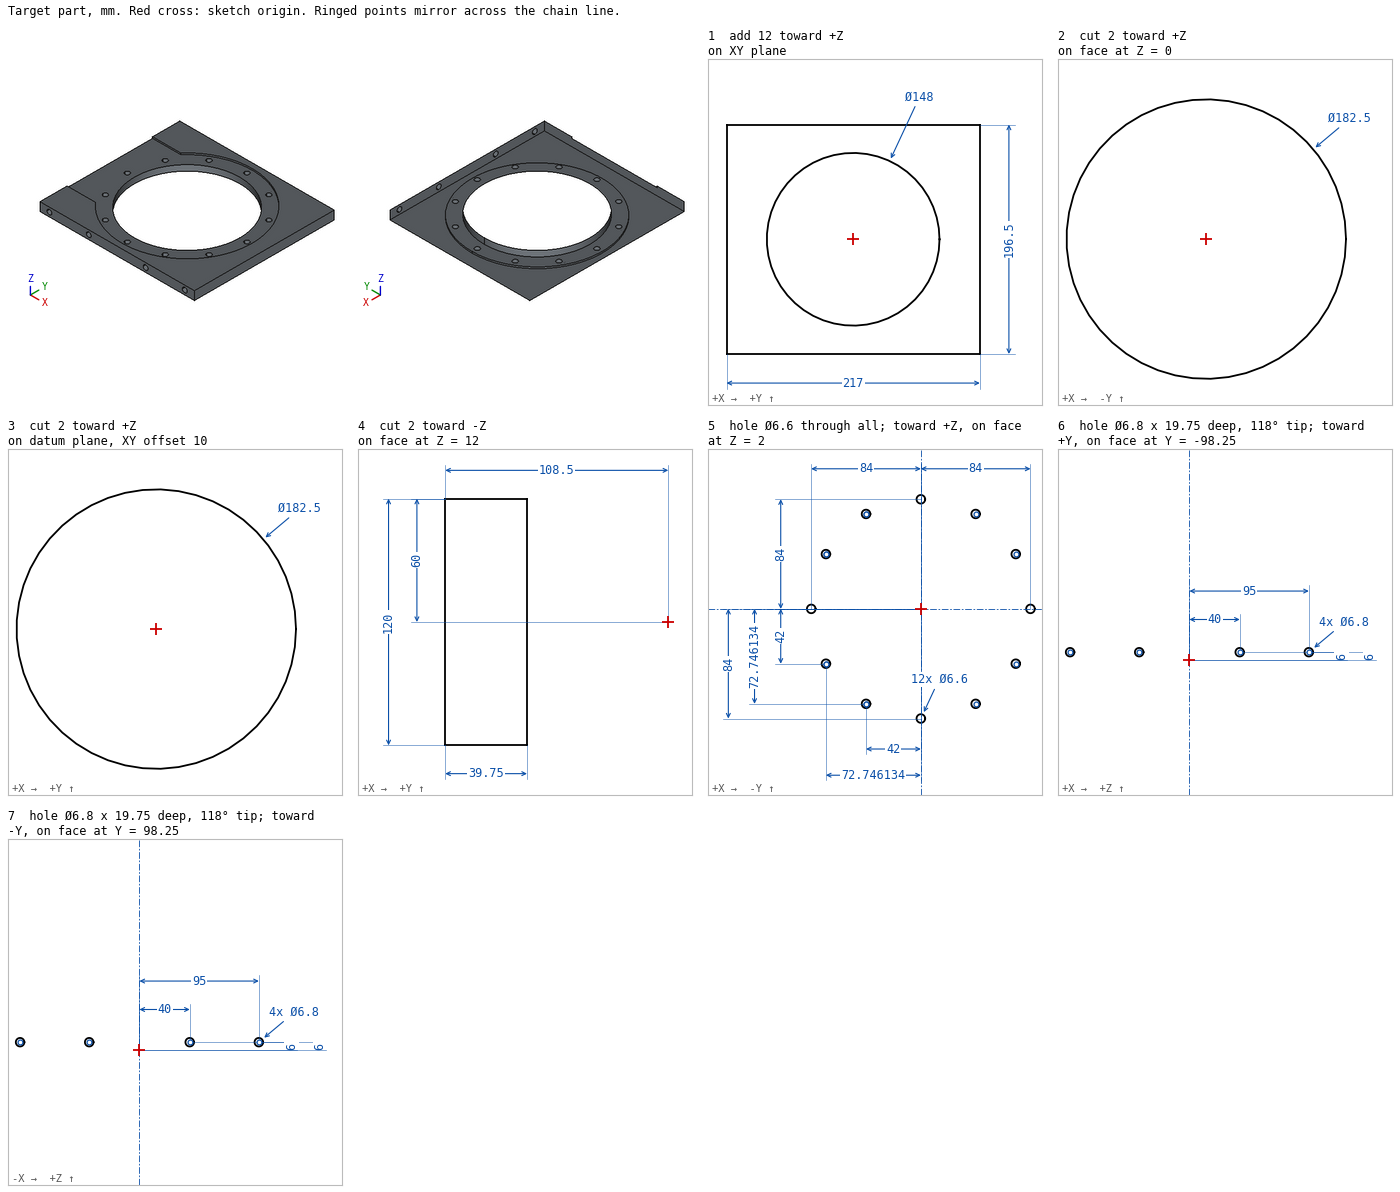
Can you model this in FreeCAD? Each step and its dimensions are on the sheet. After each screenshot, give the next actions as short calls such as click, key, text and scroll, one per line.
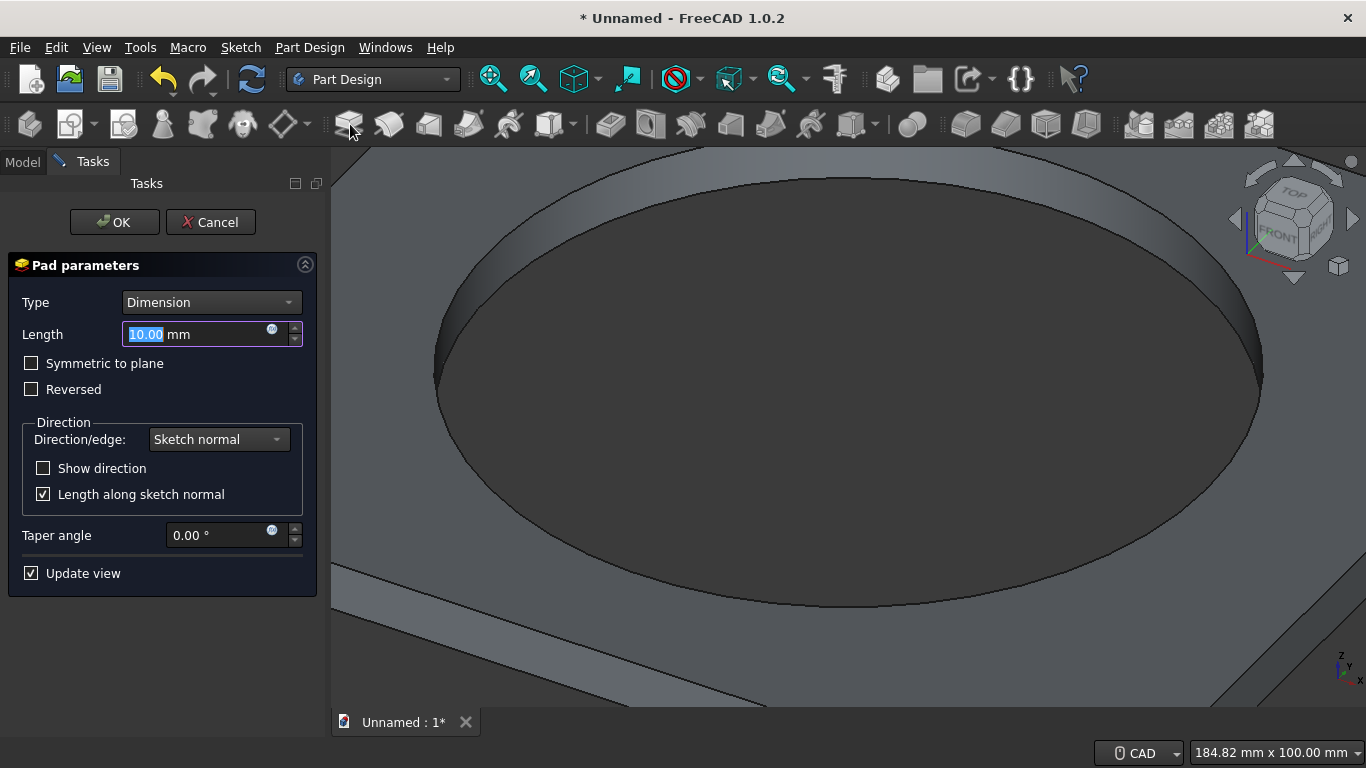
text(12)
key(Tab)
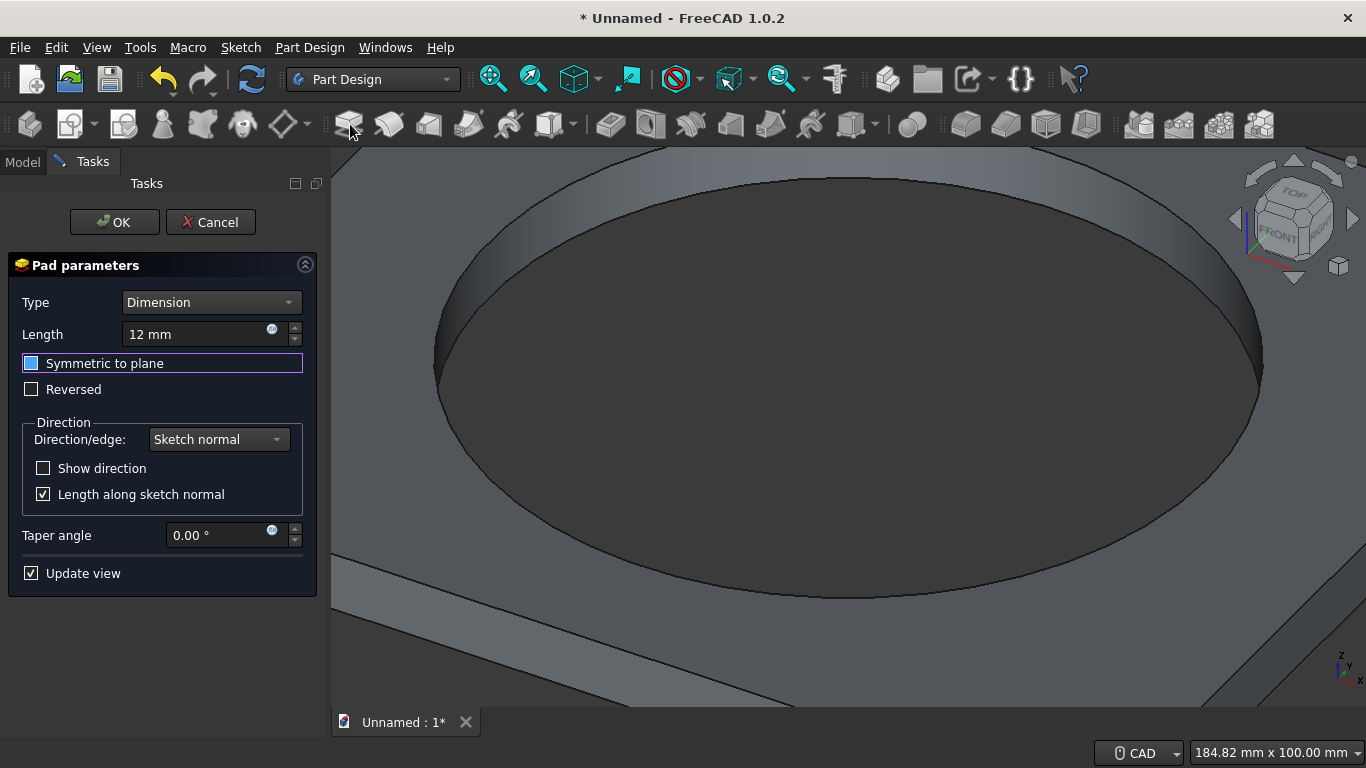
click(115, 222)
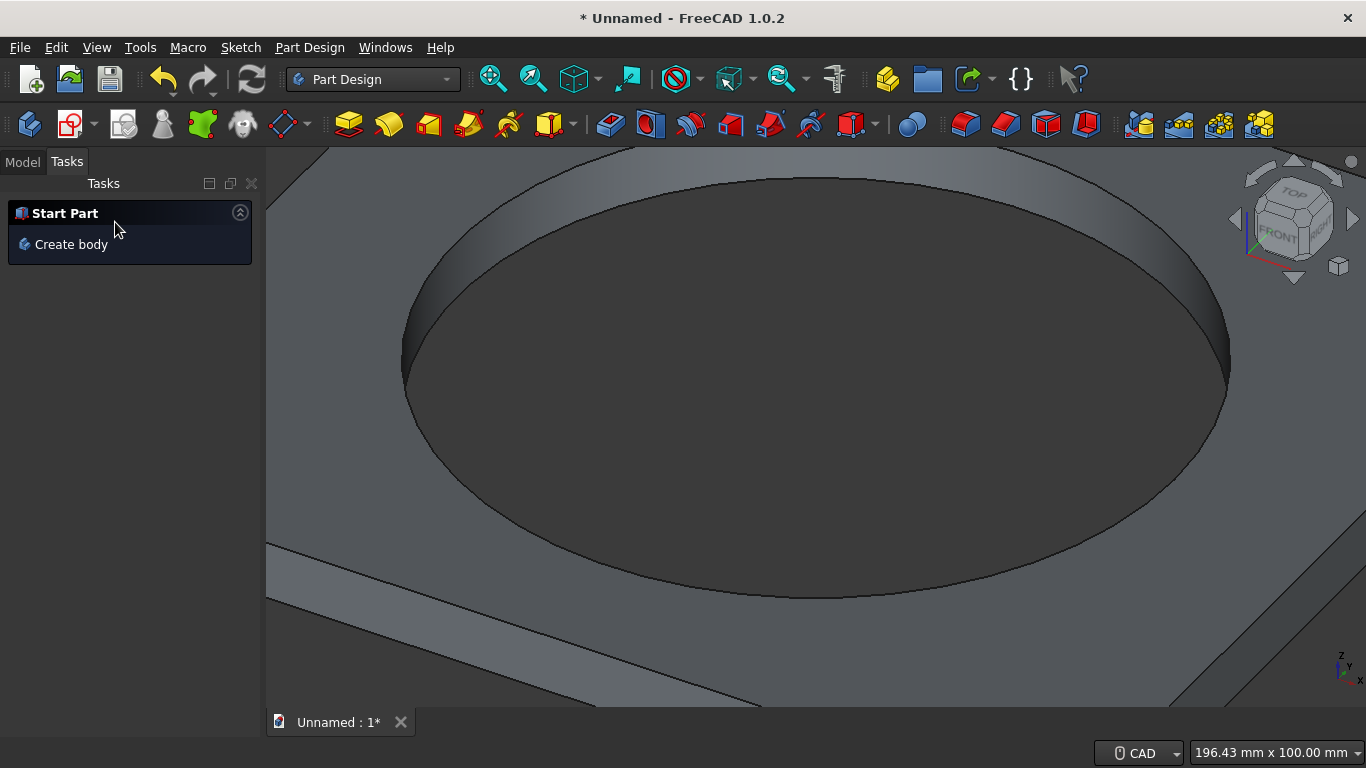
click(494, 80)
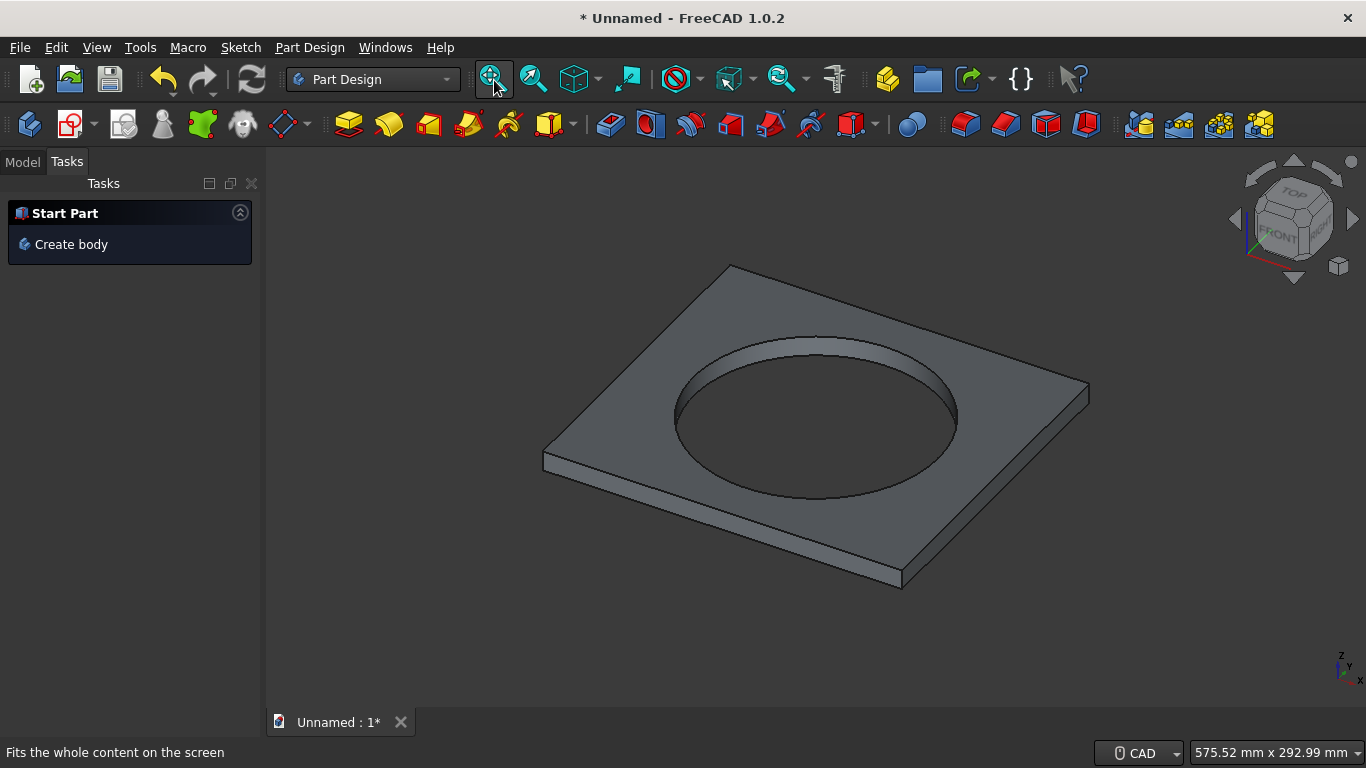
key(5)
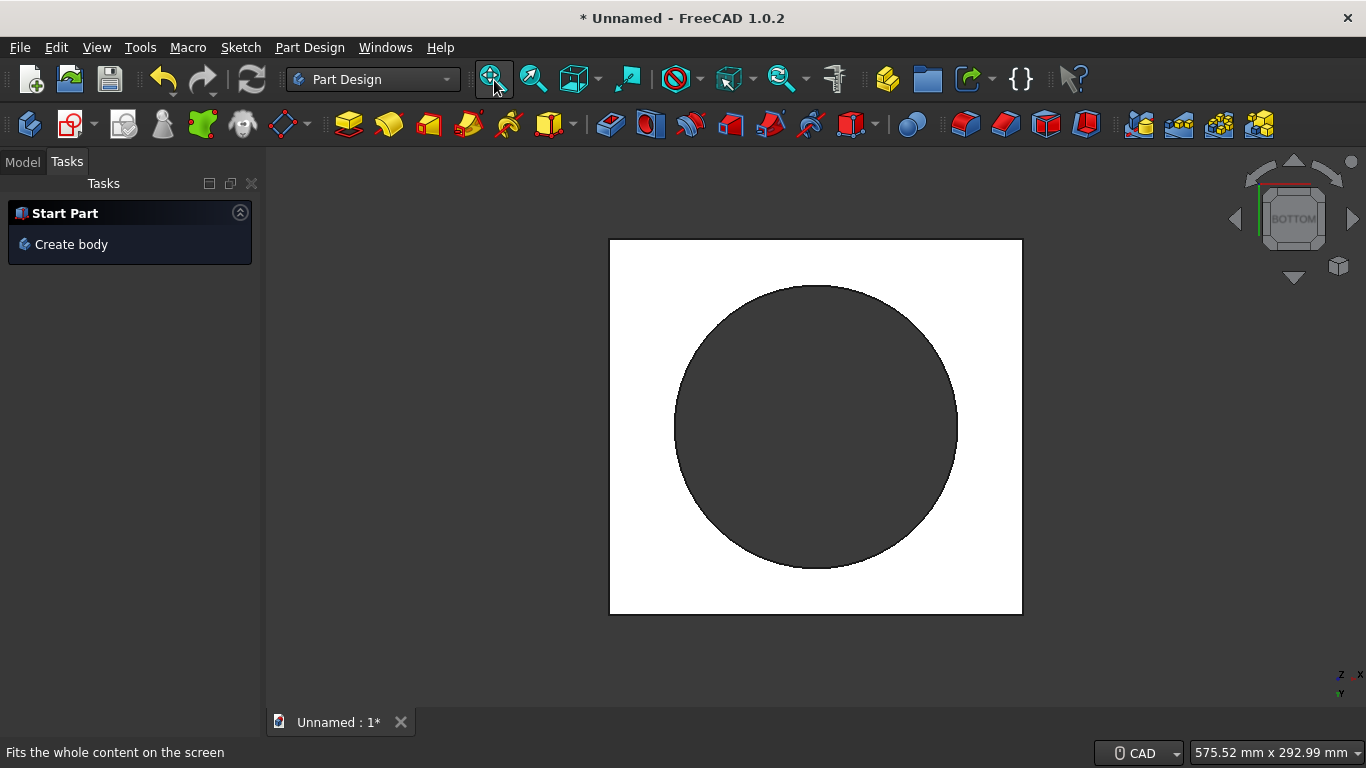
click(994, 533)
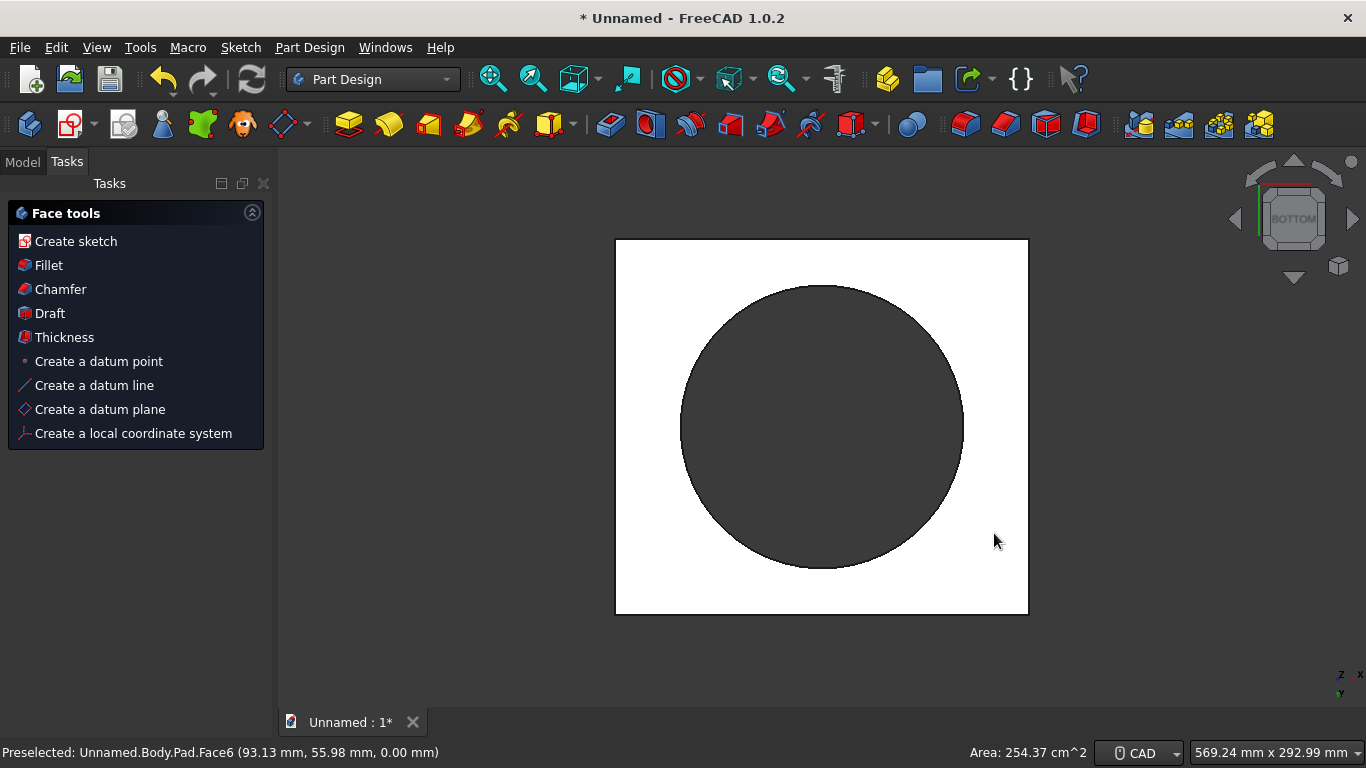
click(70, 124)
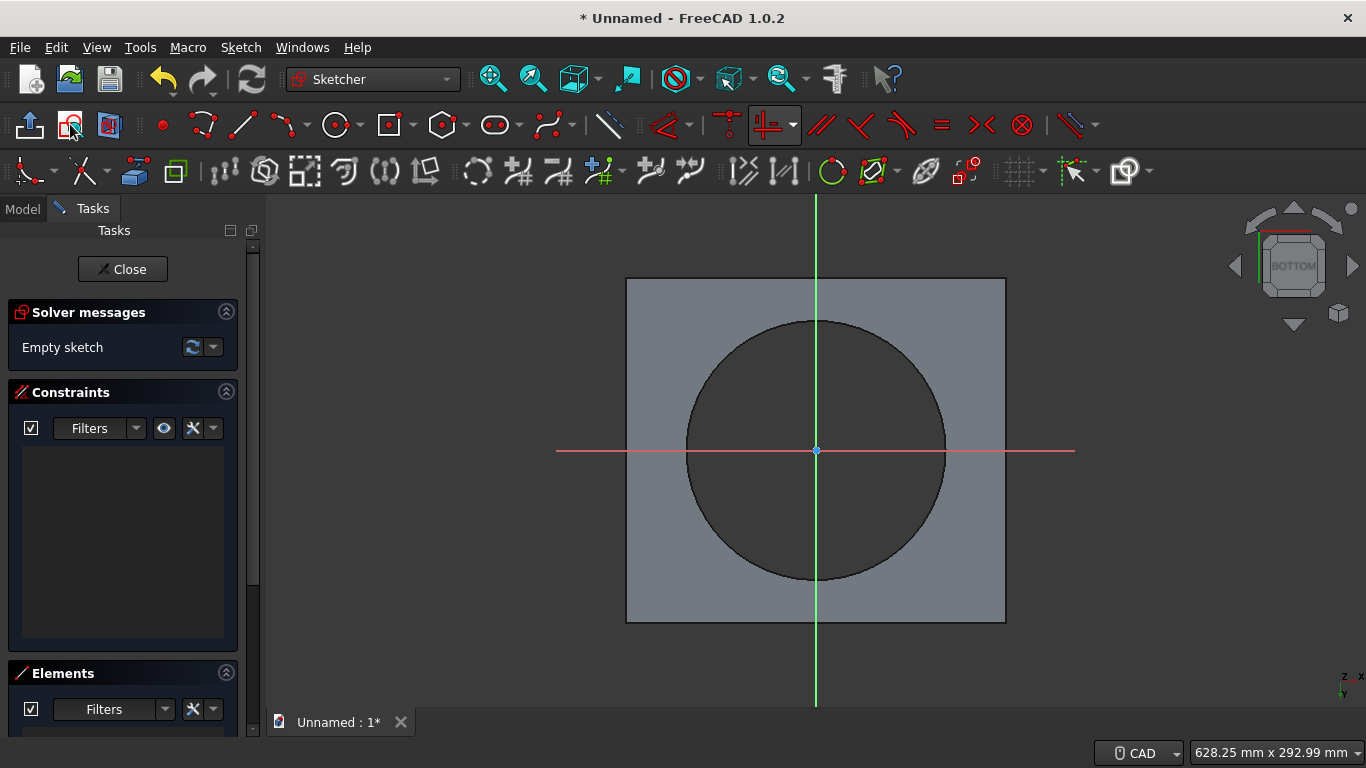
click(336, 126)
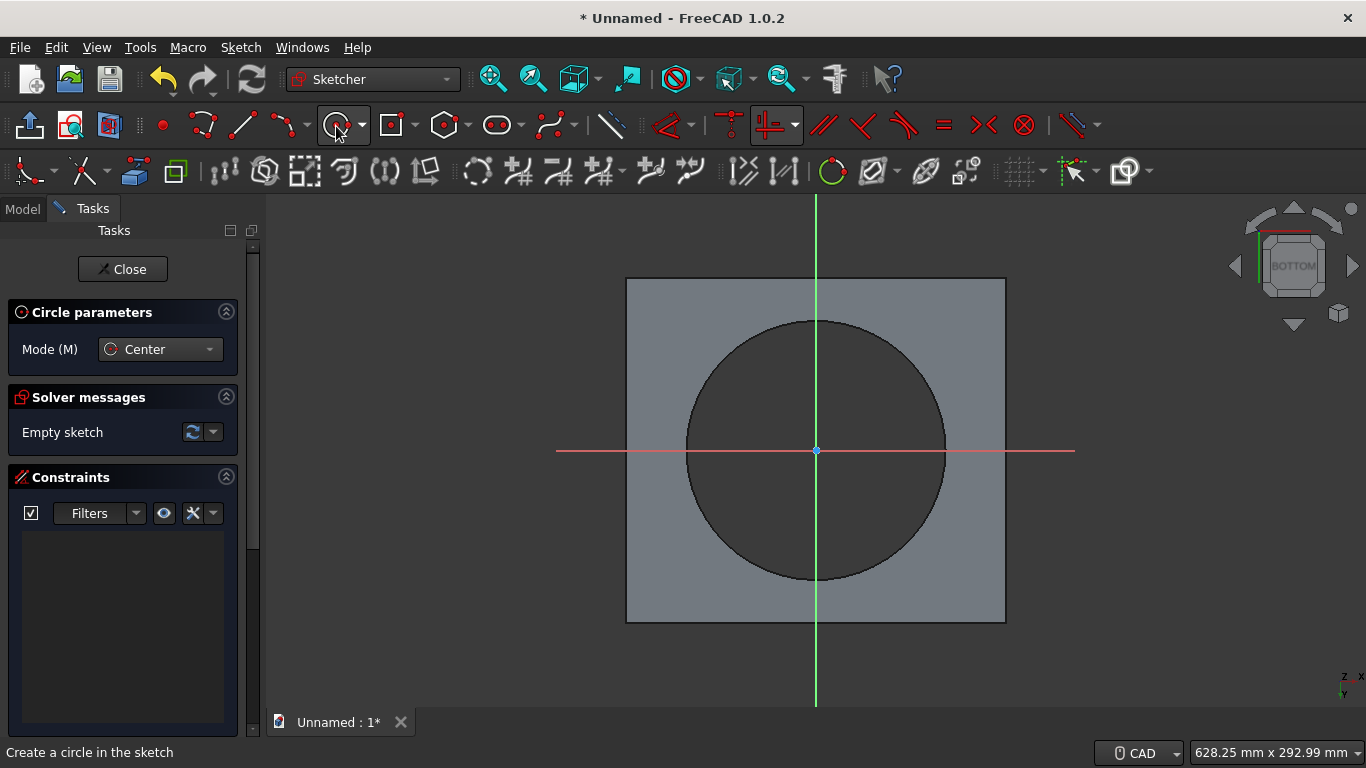
click(816, 450)
click(929, 338)
key(Escape)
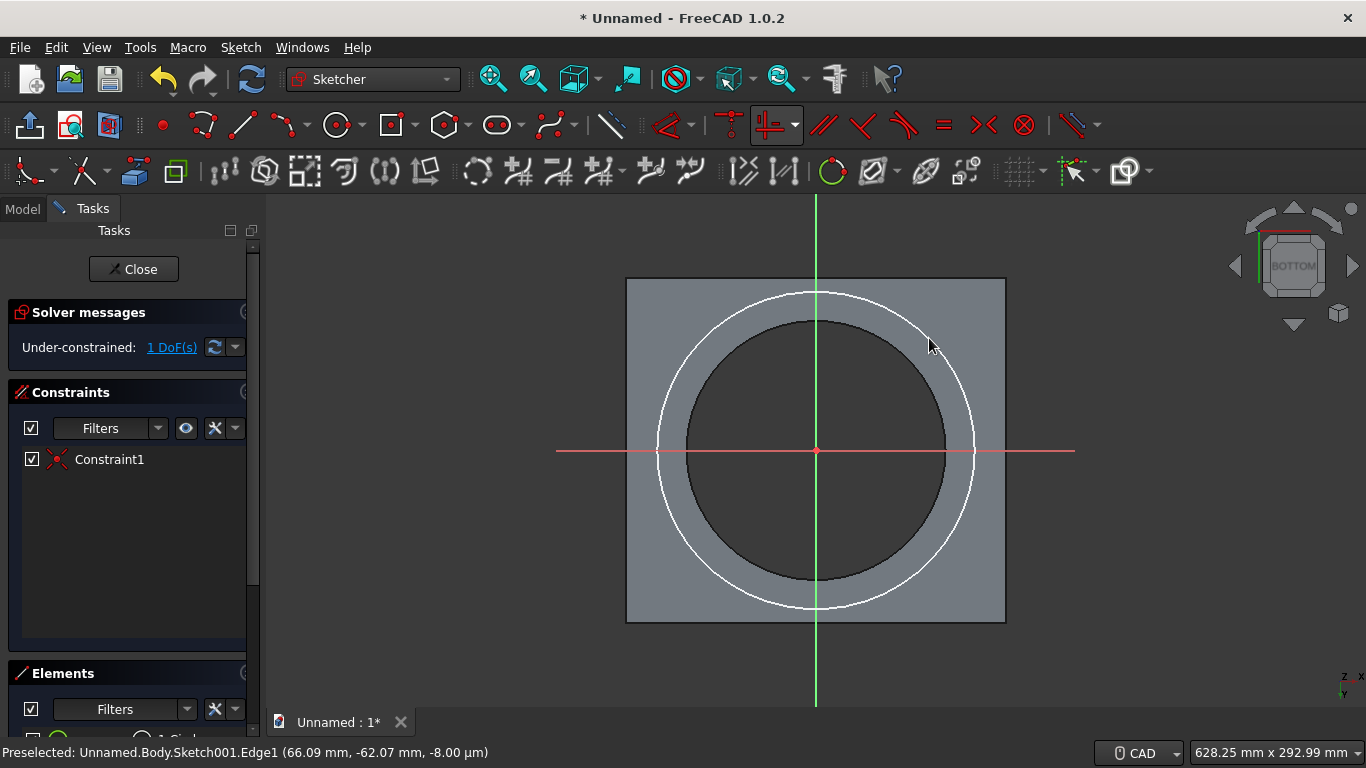
click(666, 126)